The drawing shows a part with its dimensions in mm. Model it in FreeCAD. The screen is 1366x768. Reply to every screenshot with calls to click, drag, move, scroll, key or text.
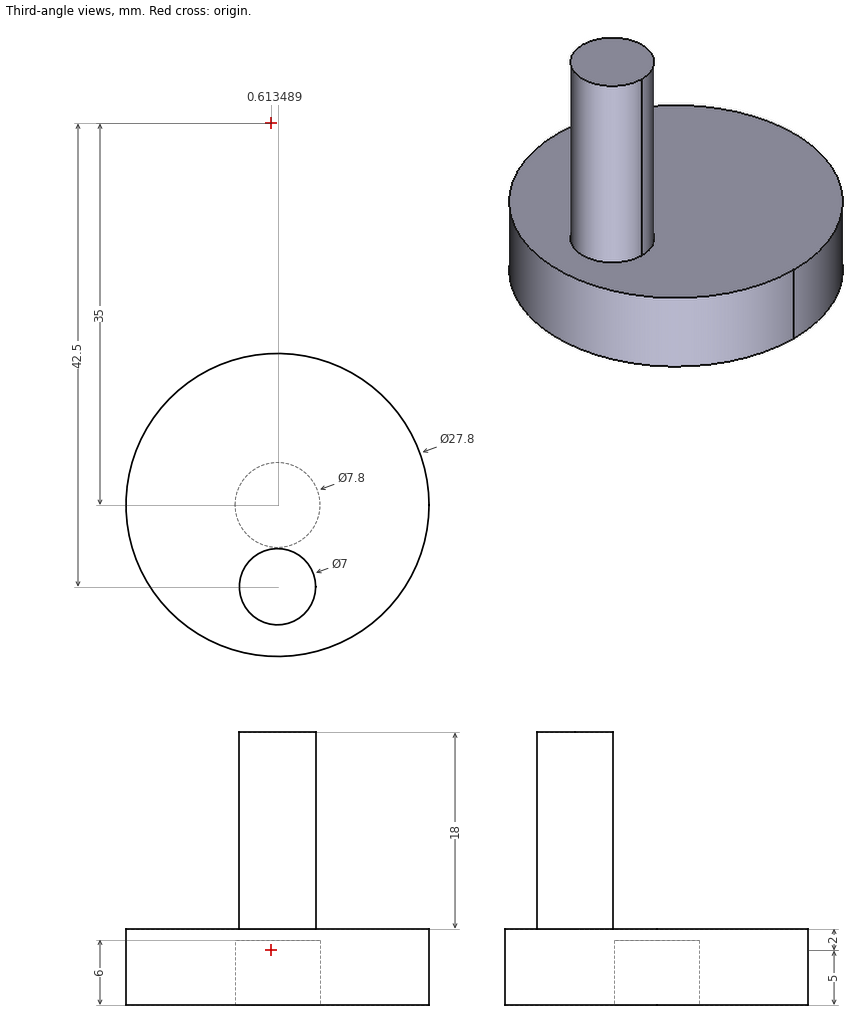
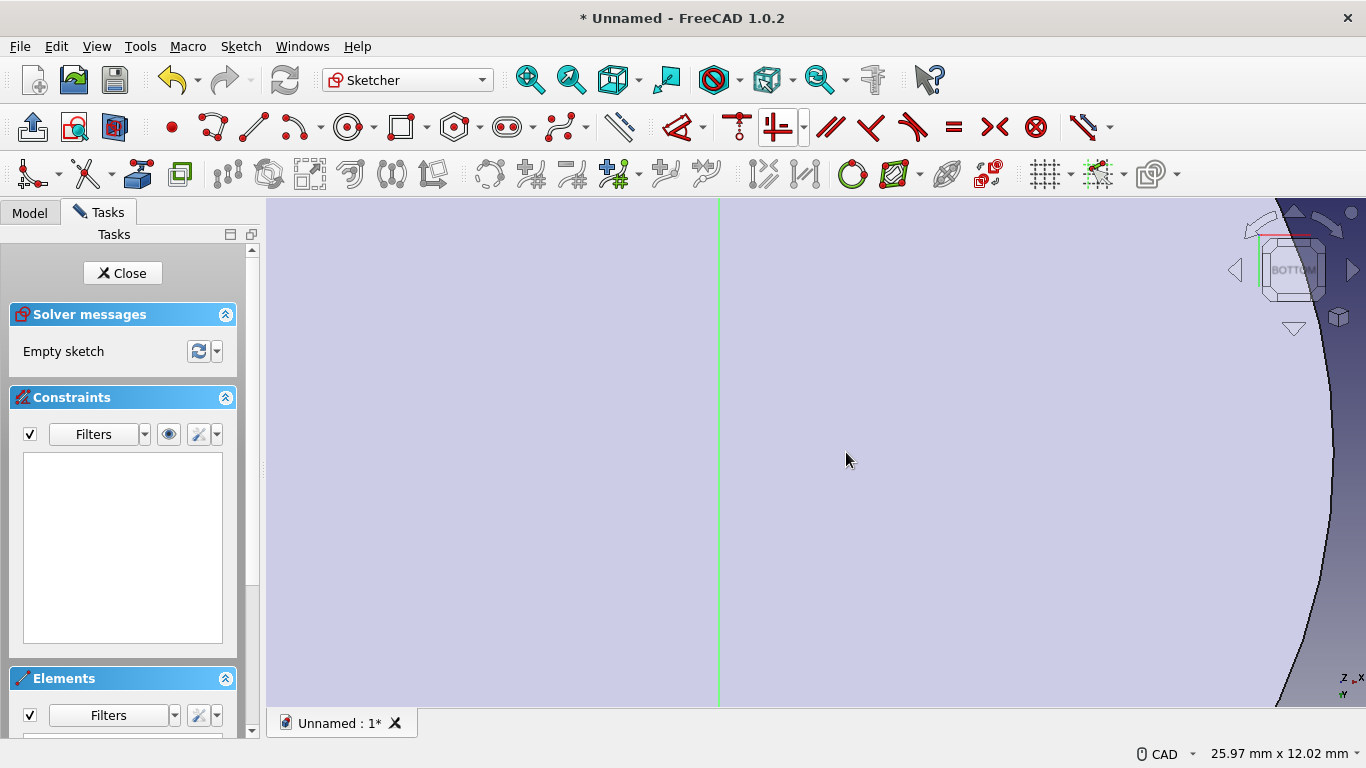
click(348, 128)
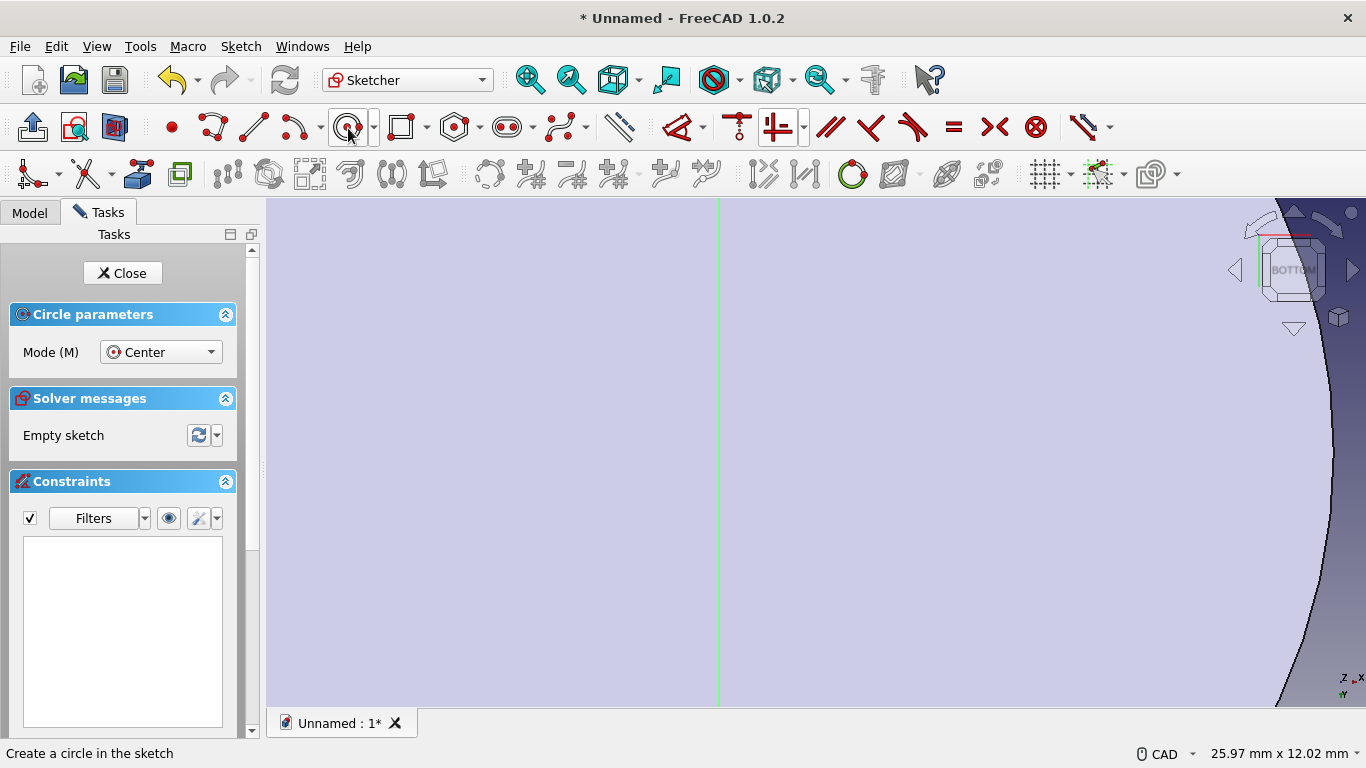
click(745, 452)
move(862, 336)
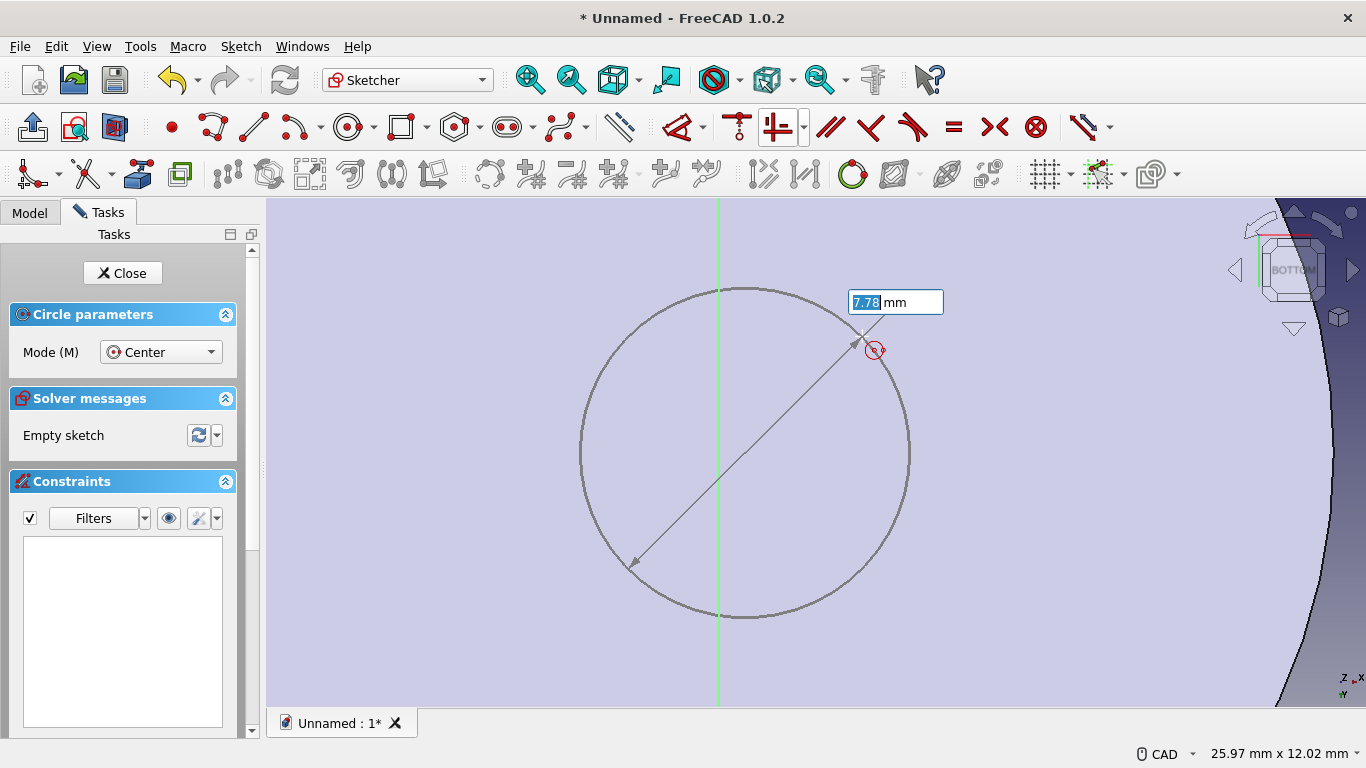
text(7.8)
key(Return)
key(Escape)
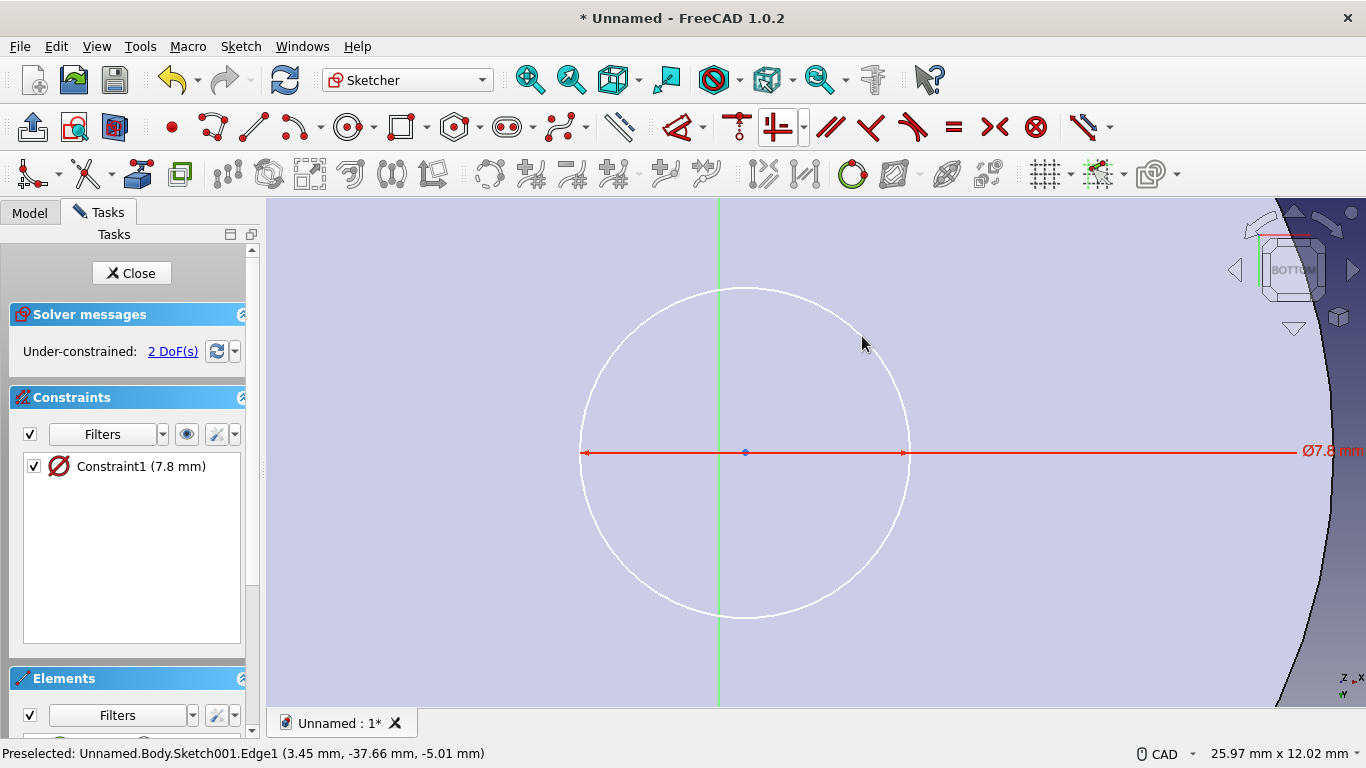
click(676, 128)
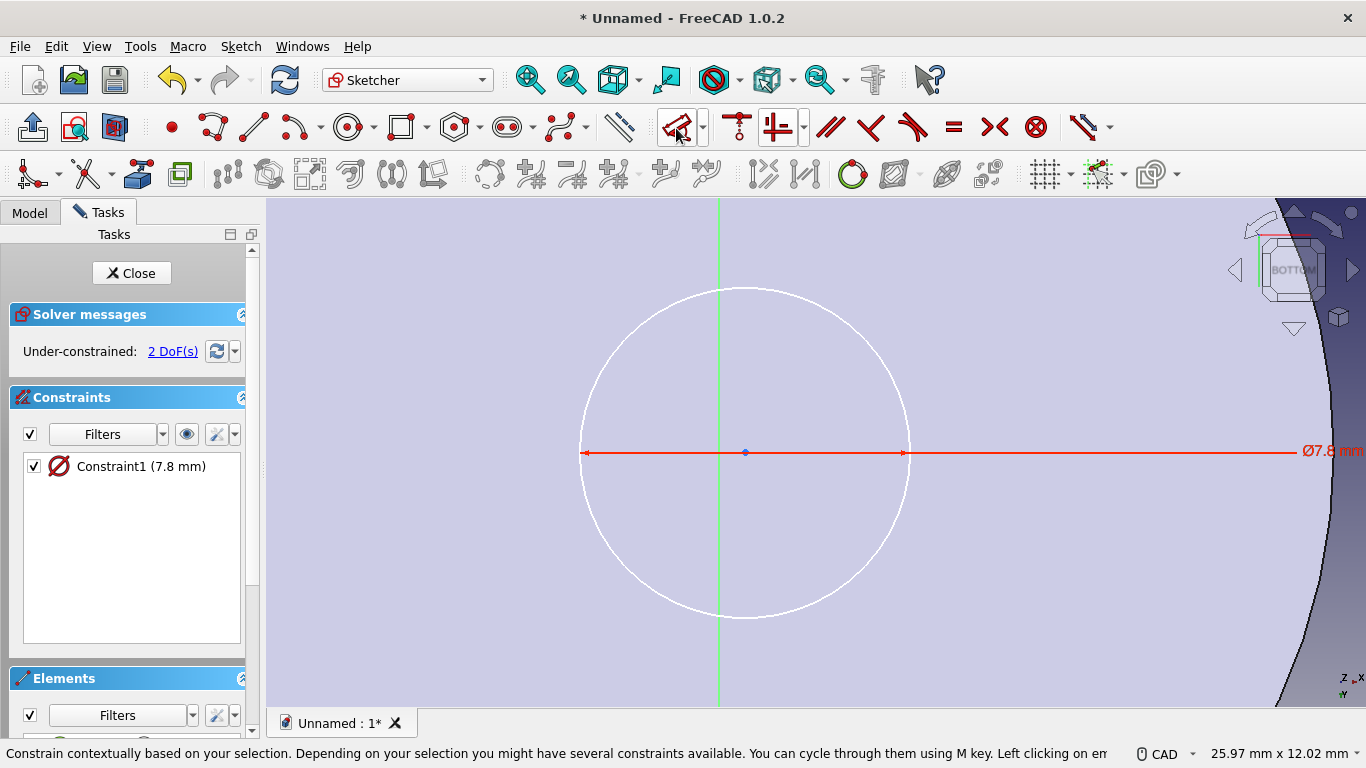
click(745, 453)
click(685, 566)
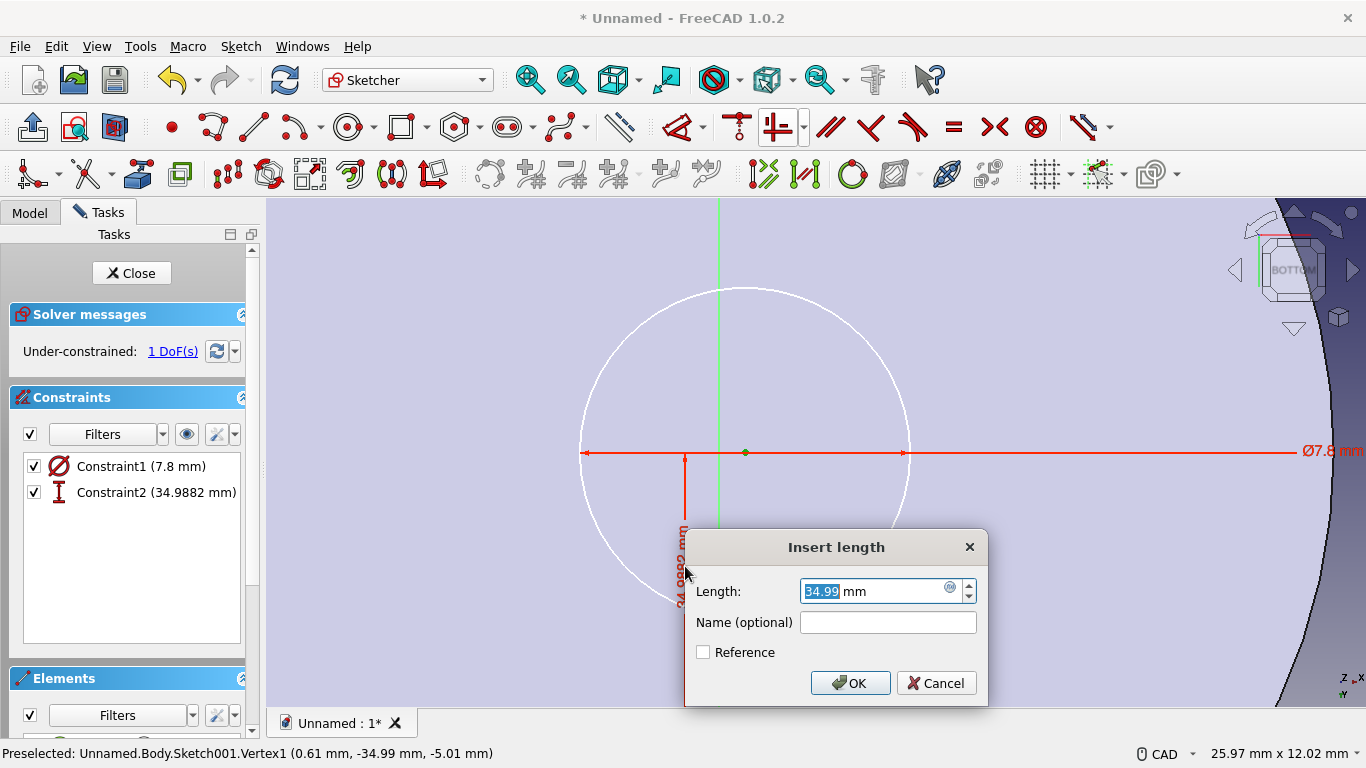
text(35)
key(Return)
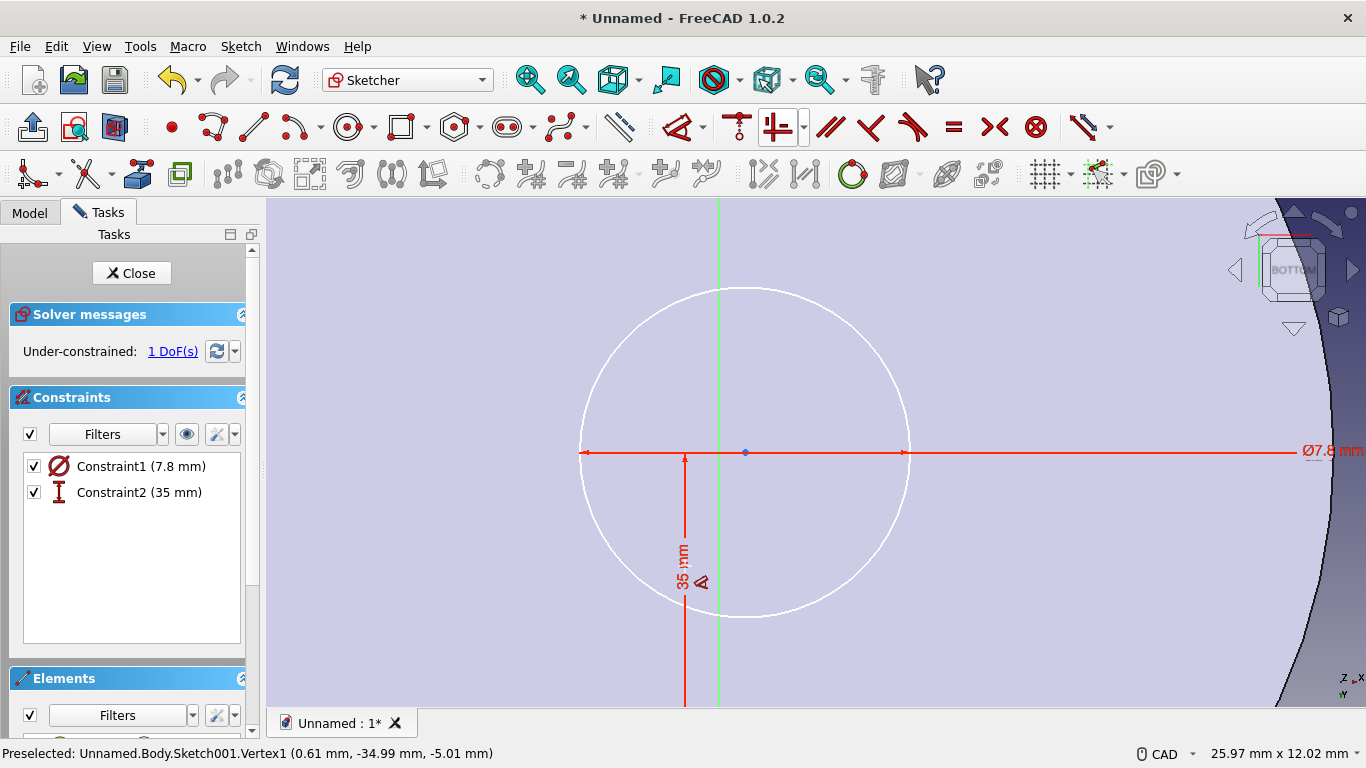
scroll(745, 452, up, 3)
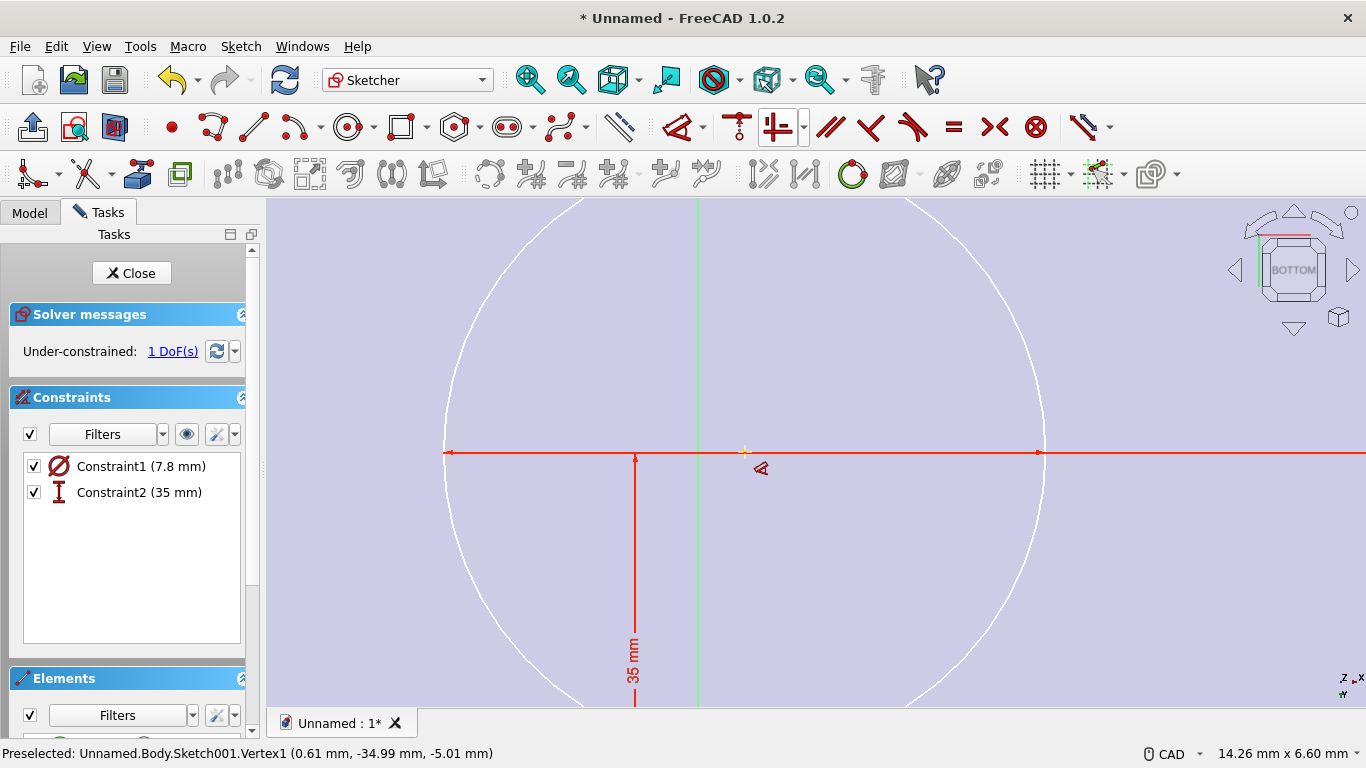
click(745, 452)
click(721, 418)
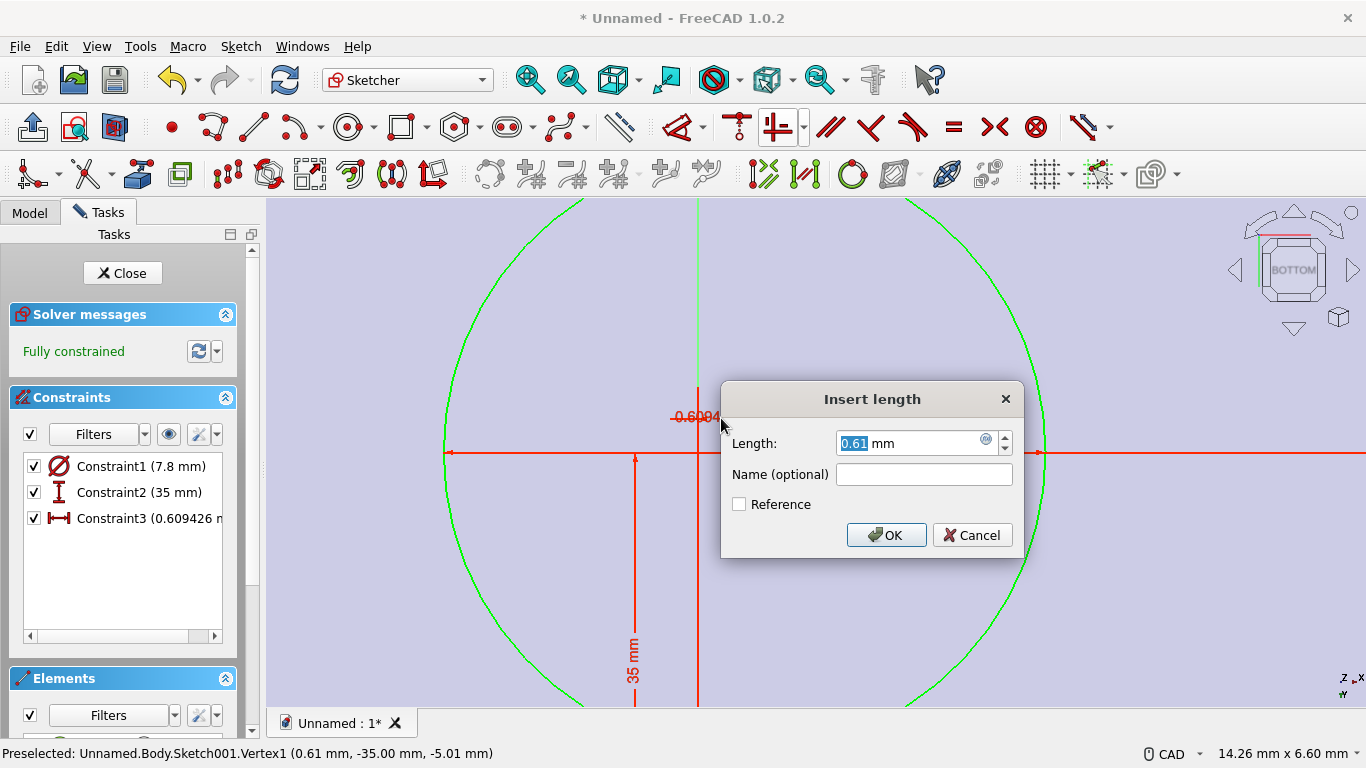
text(0.613489)
key(Return)
key(Escape)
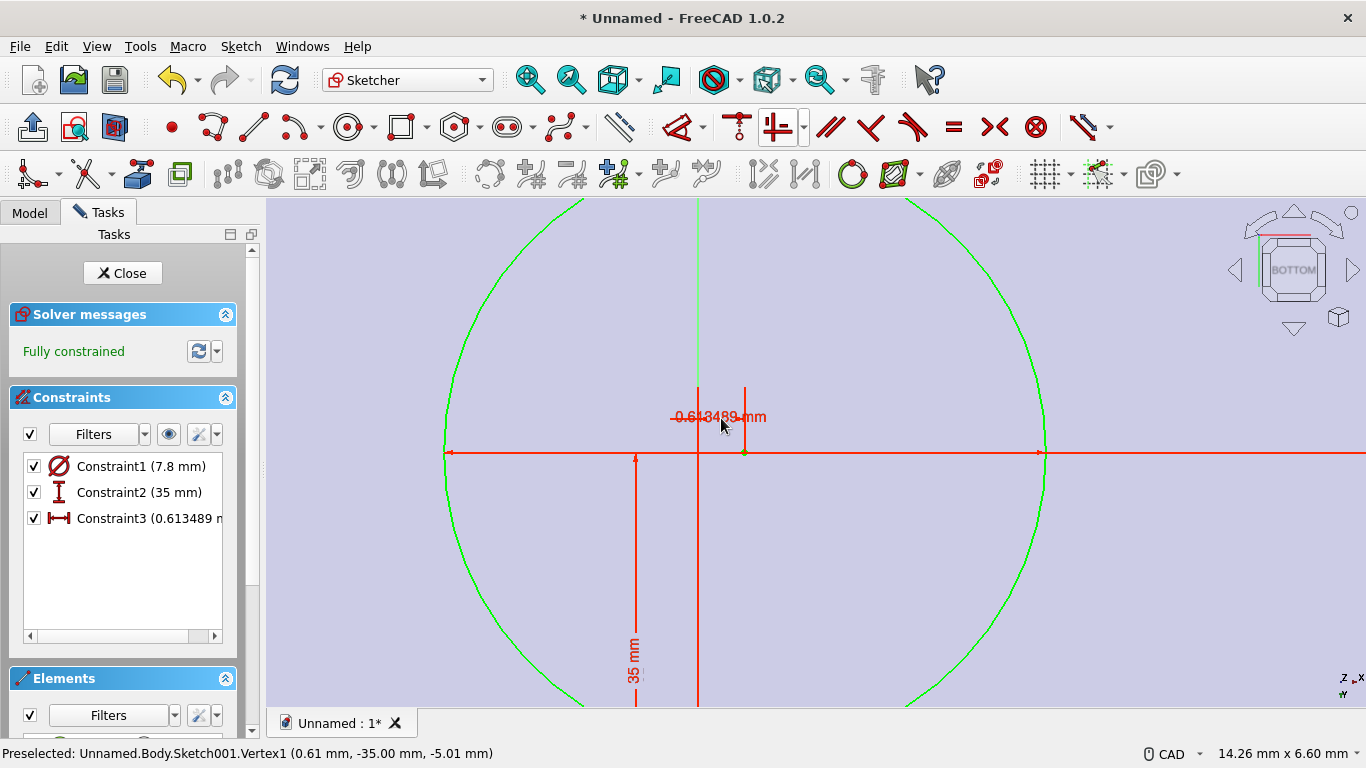
click(123, 273)